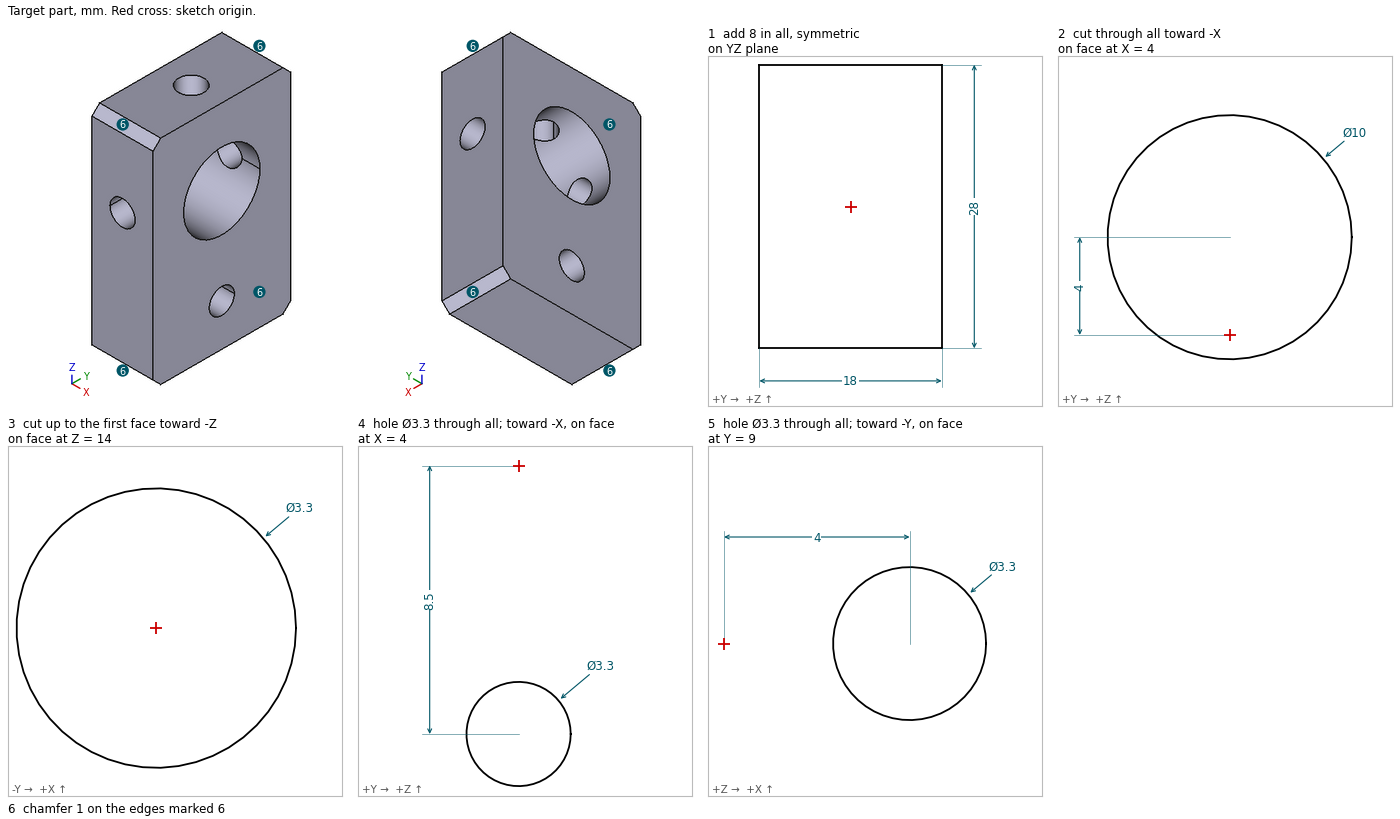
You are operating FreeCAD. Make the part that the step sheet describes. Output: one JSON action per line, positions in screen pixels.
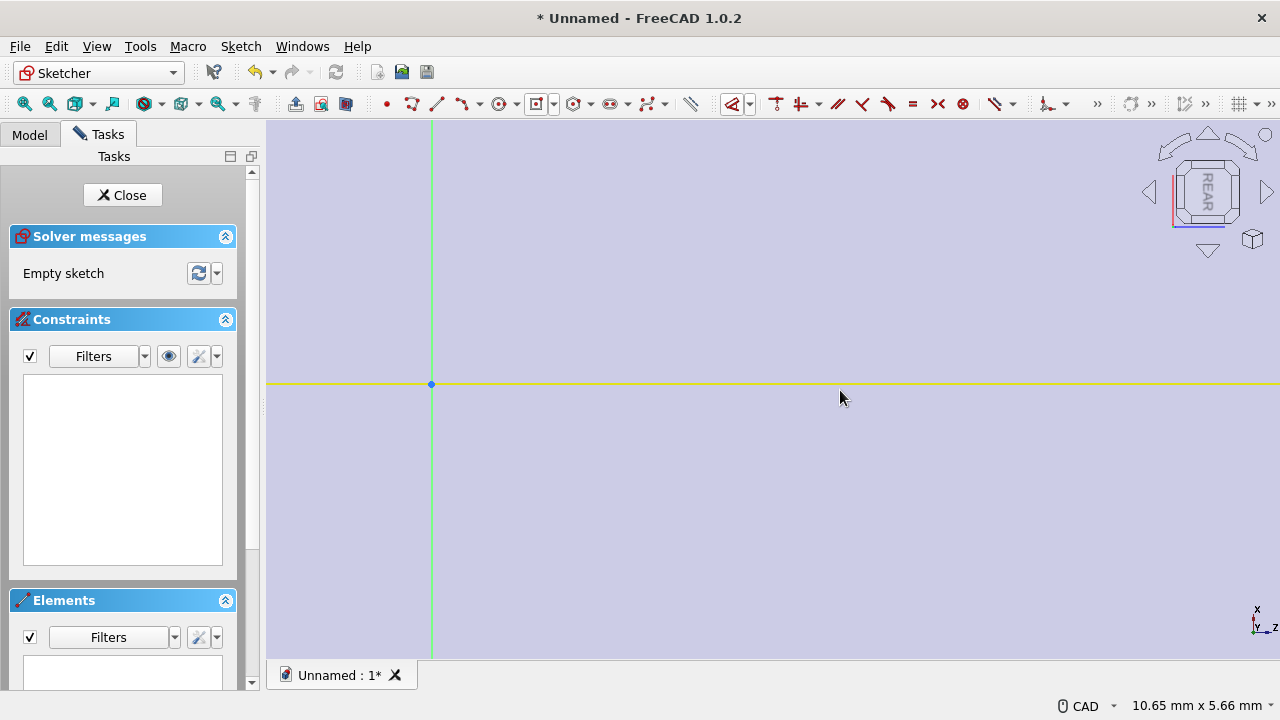
{"action": "left_click", "coordinate": [498, 104]}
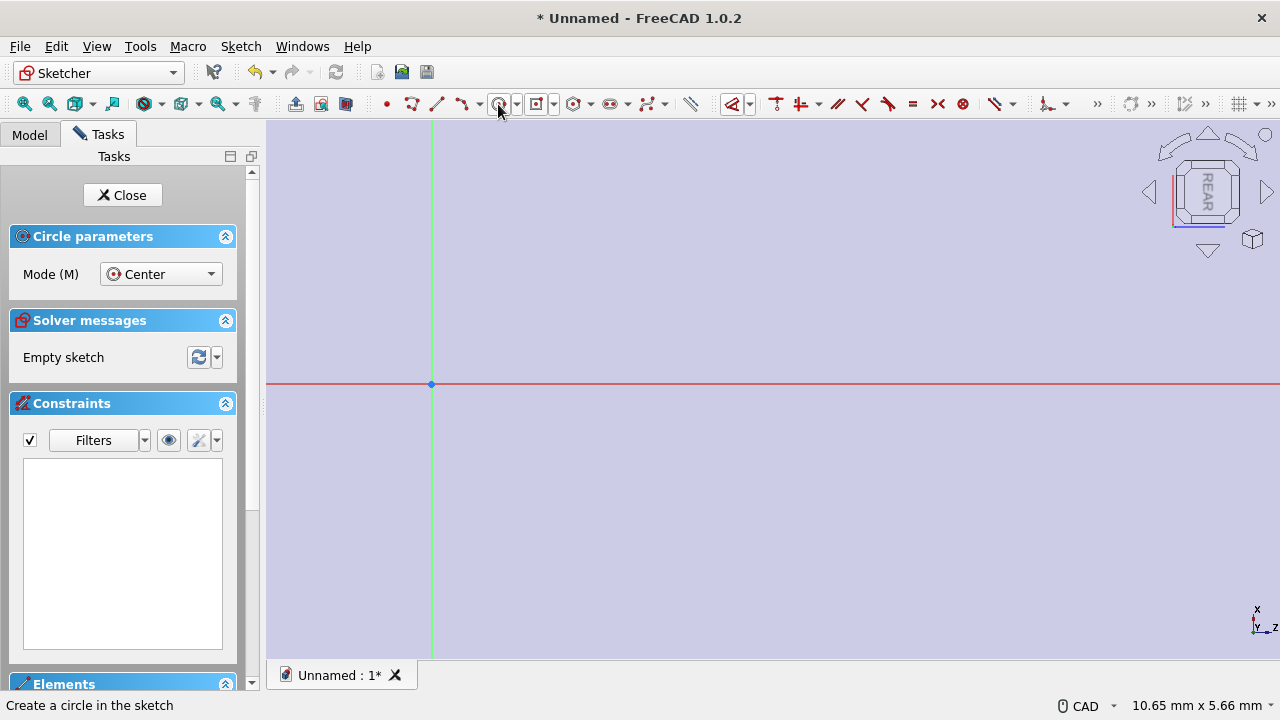
{"action": "left_click", "coordinate": [813, 384]}
{"action": "left_click", "coordinate": [924, 273]}
{"action": "key", "text": "Escape"}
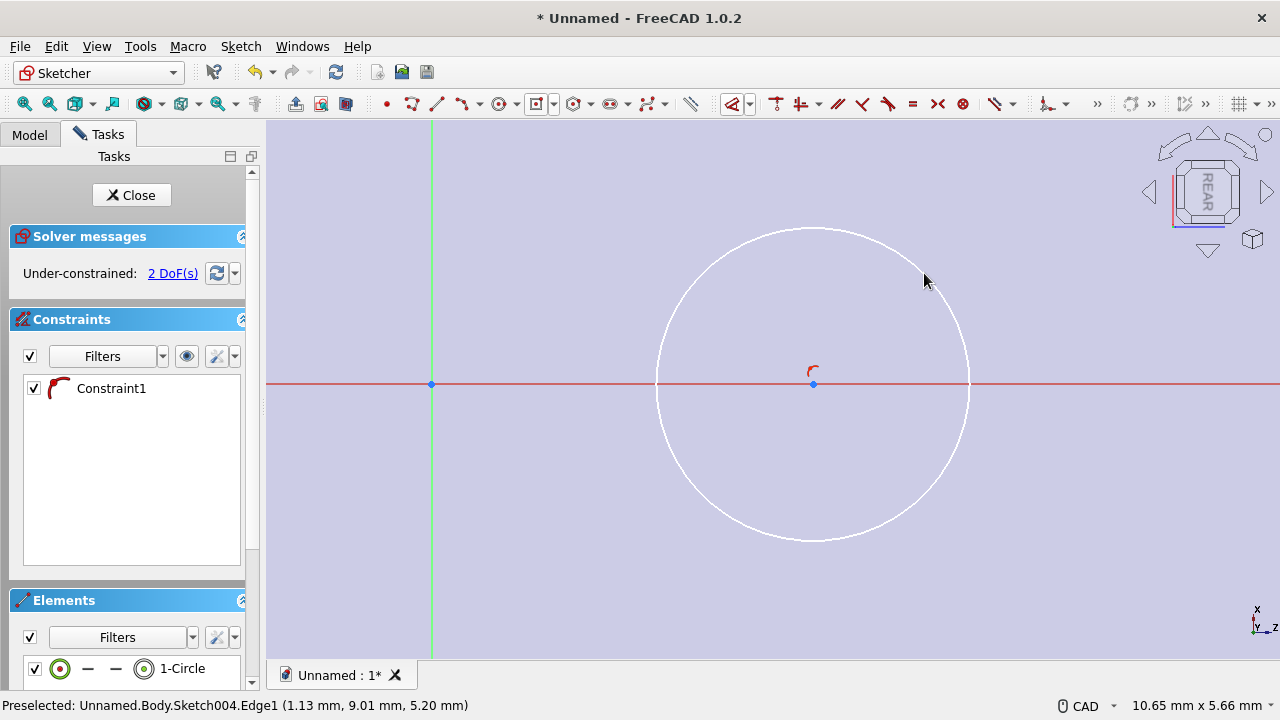
{"action": "left_click", "coordinate": [923, 273]}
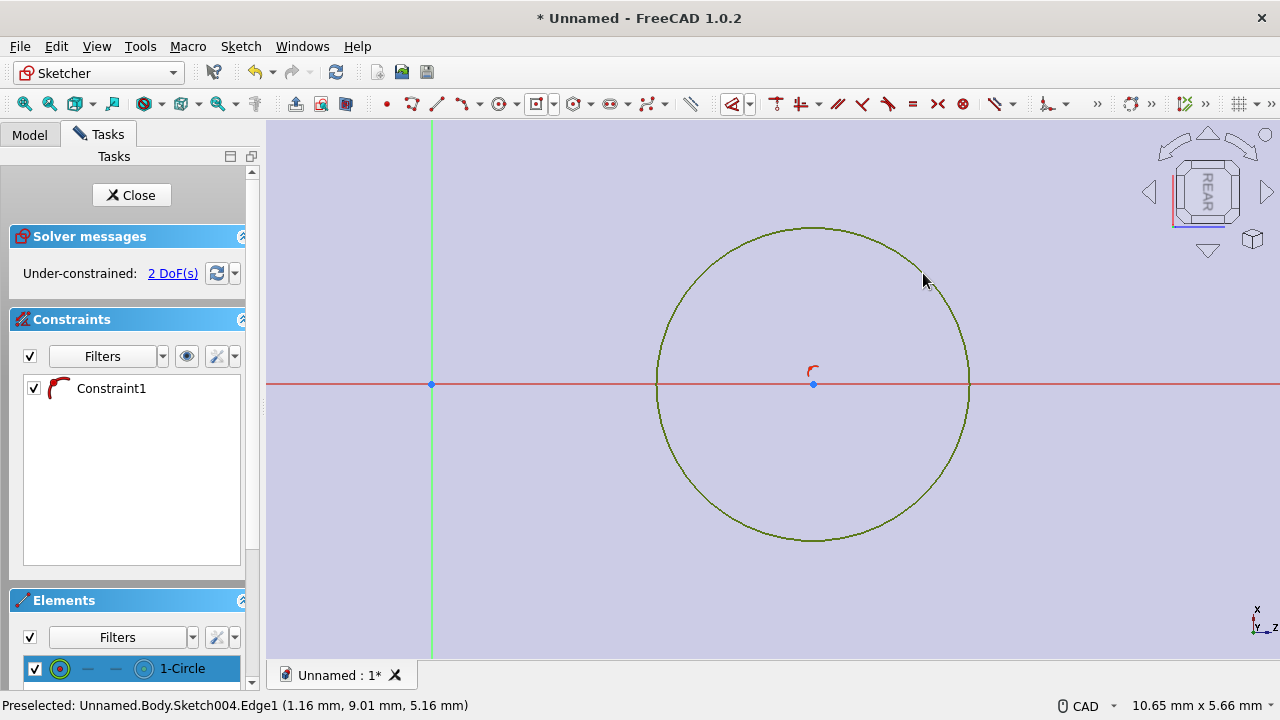
{"action": "key", "text": "k o"}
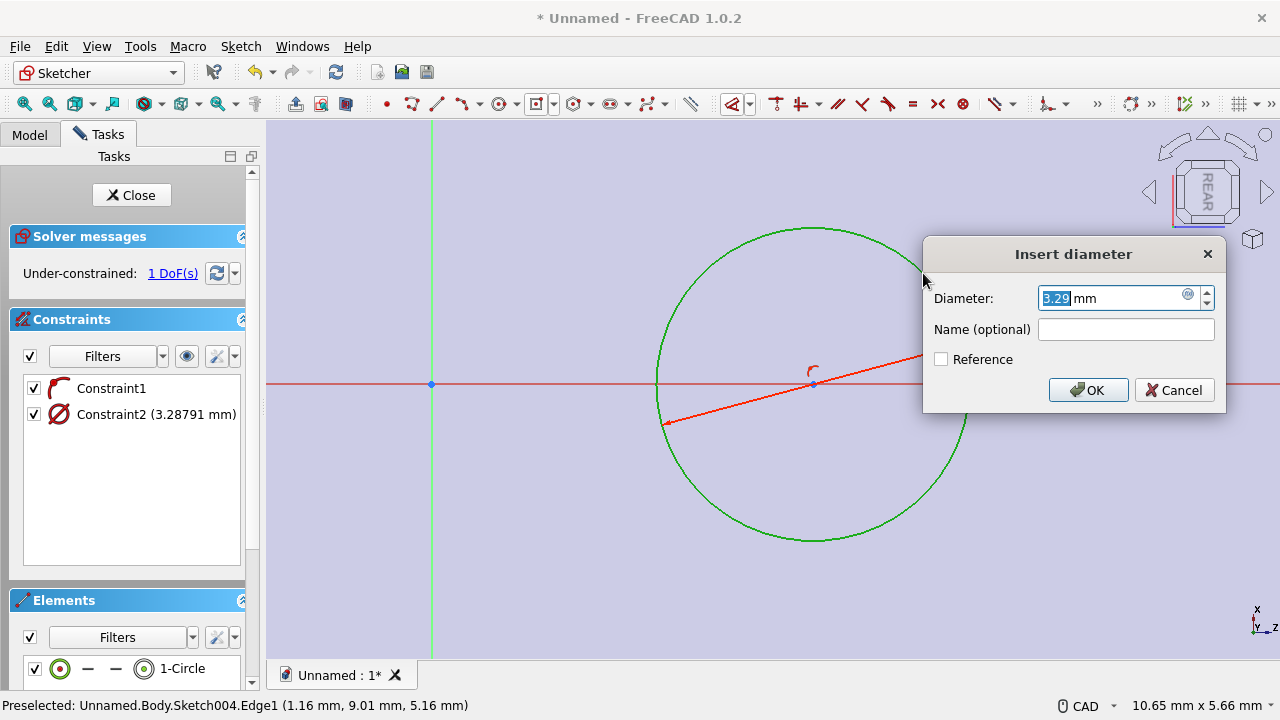
{"action": "type", "text": "3.3"}
{"action": "key", "text": "Return"}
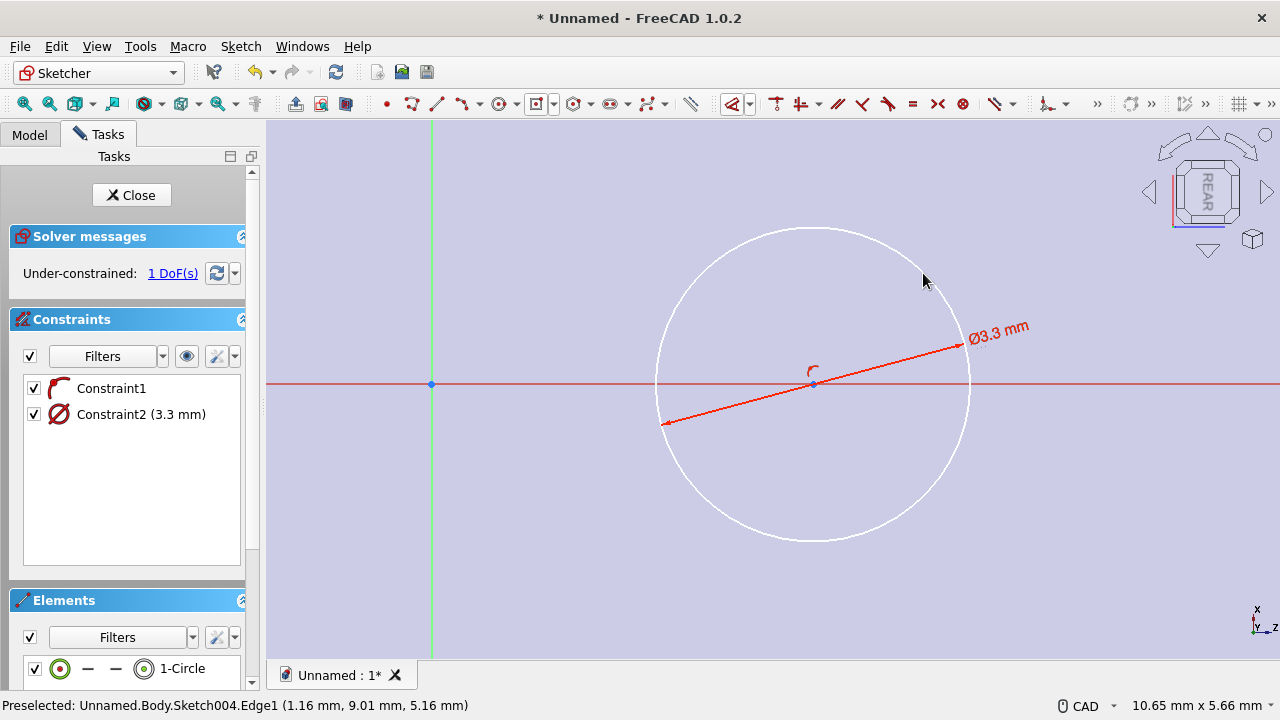
{"action": "left_click", "coordinate": [813, 384]}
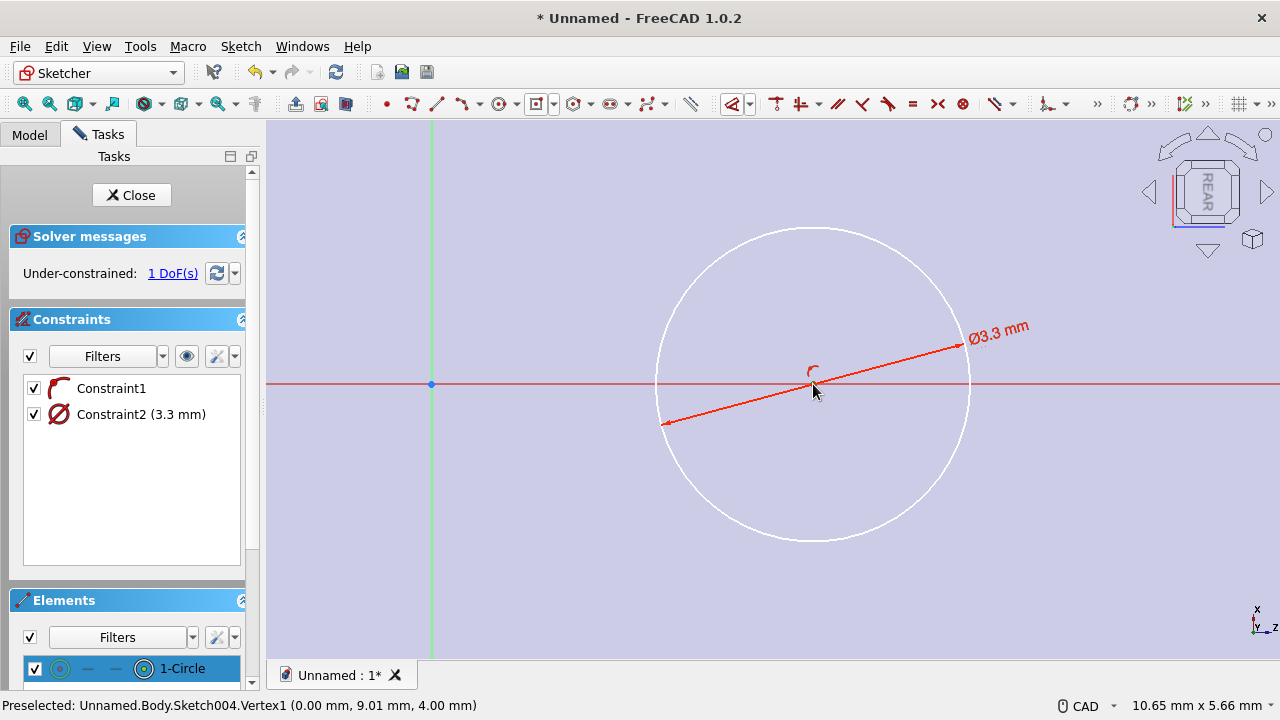
{"action": "key", "text": "l"}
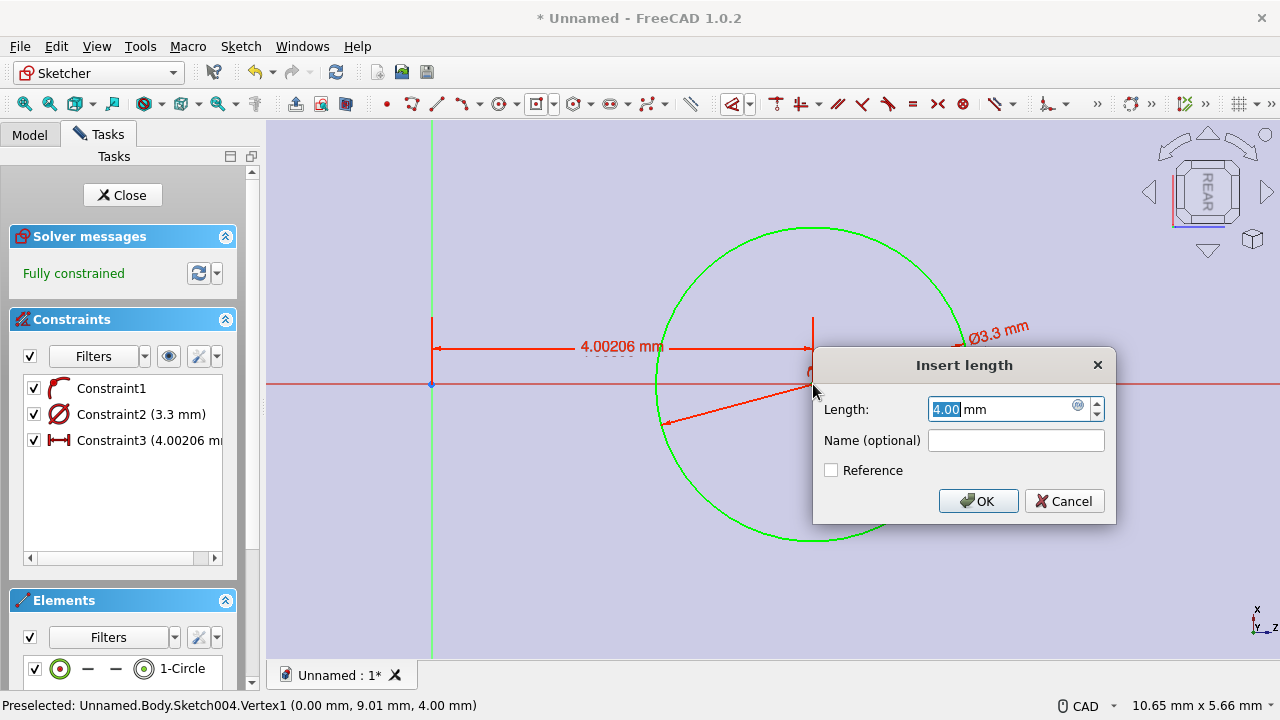
{"action": "type", "text": "4"}
{"action": "key", "text": "Return"}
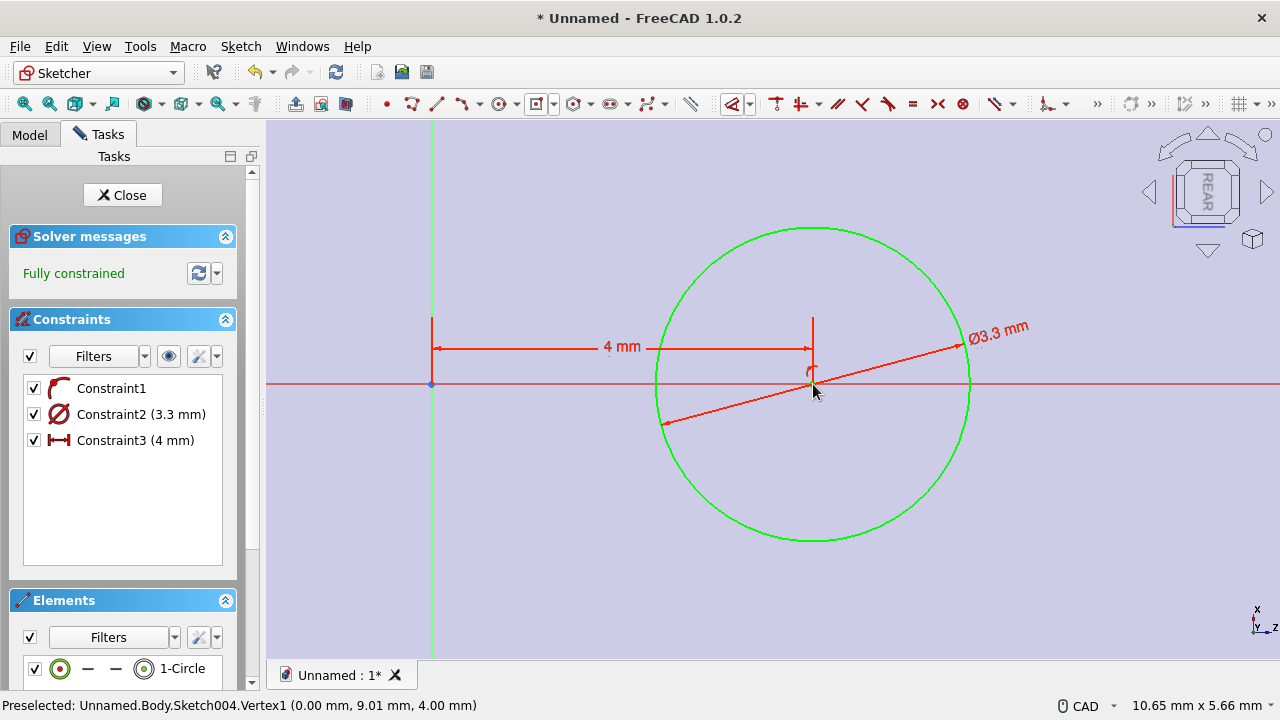
{"action": "left_click", "coordinate": [123, 195]}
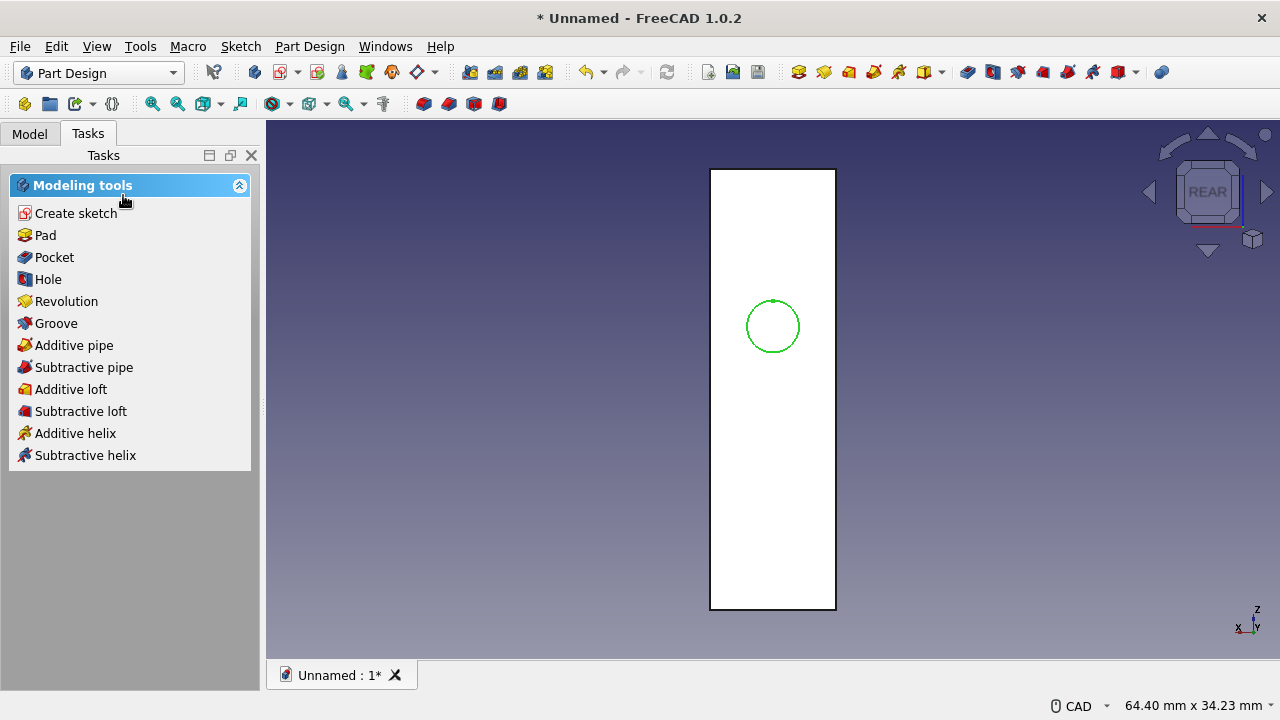
{"action": "left_click", "coordinate": [993, 72]}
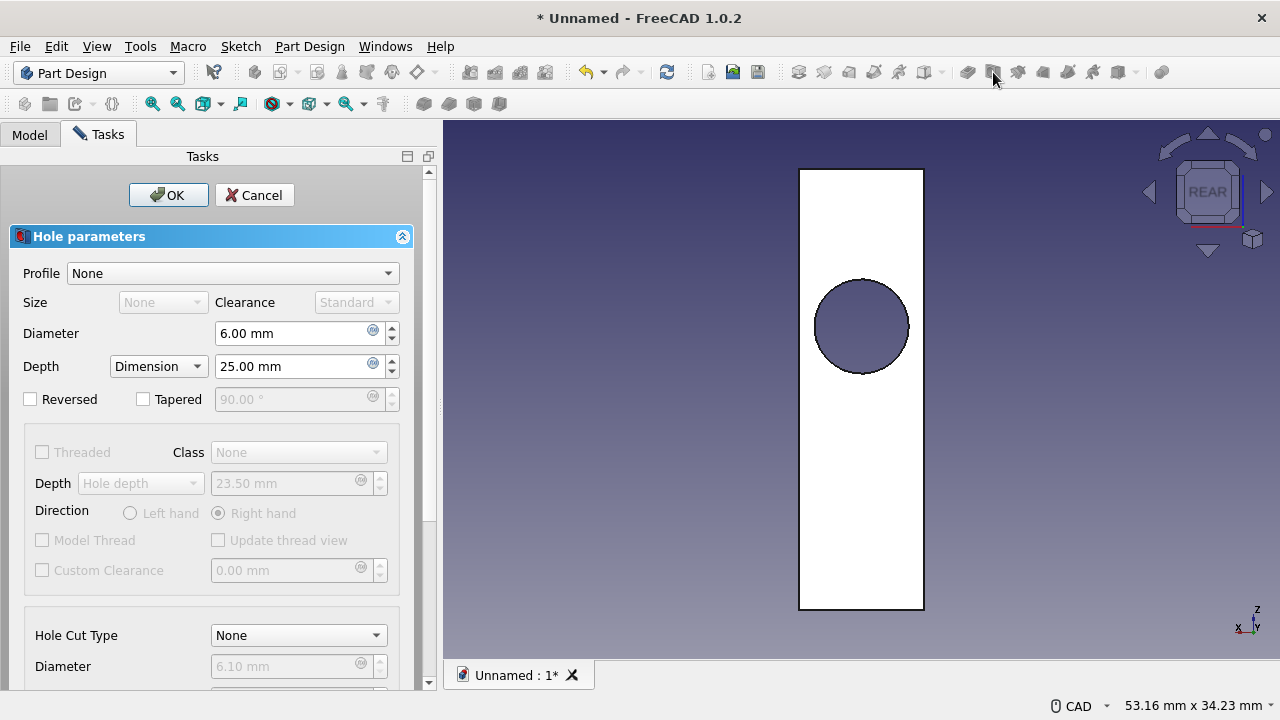
{"action": "triple_click", "coordinate": [300, 334]}